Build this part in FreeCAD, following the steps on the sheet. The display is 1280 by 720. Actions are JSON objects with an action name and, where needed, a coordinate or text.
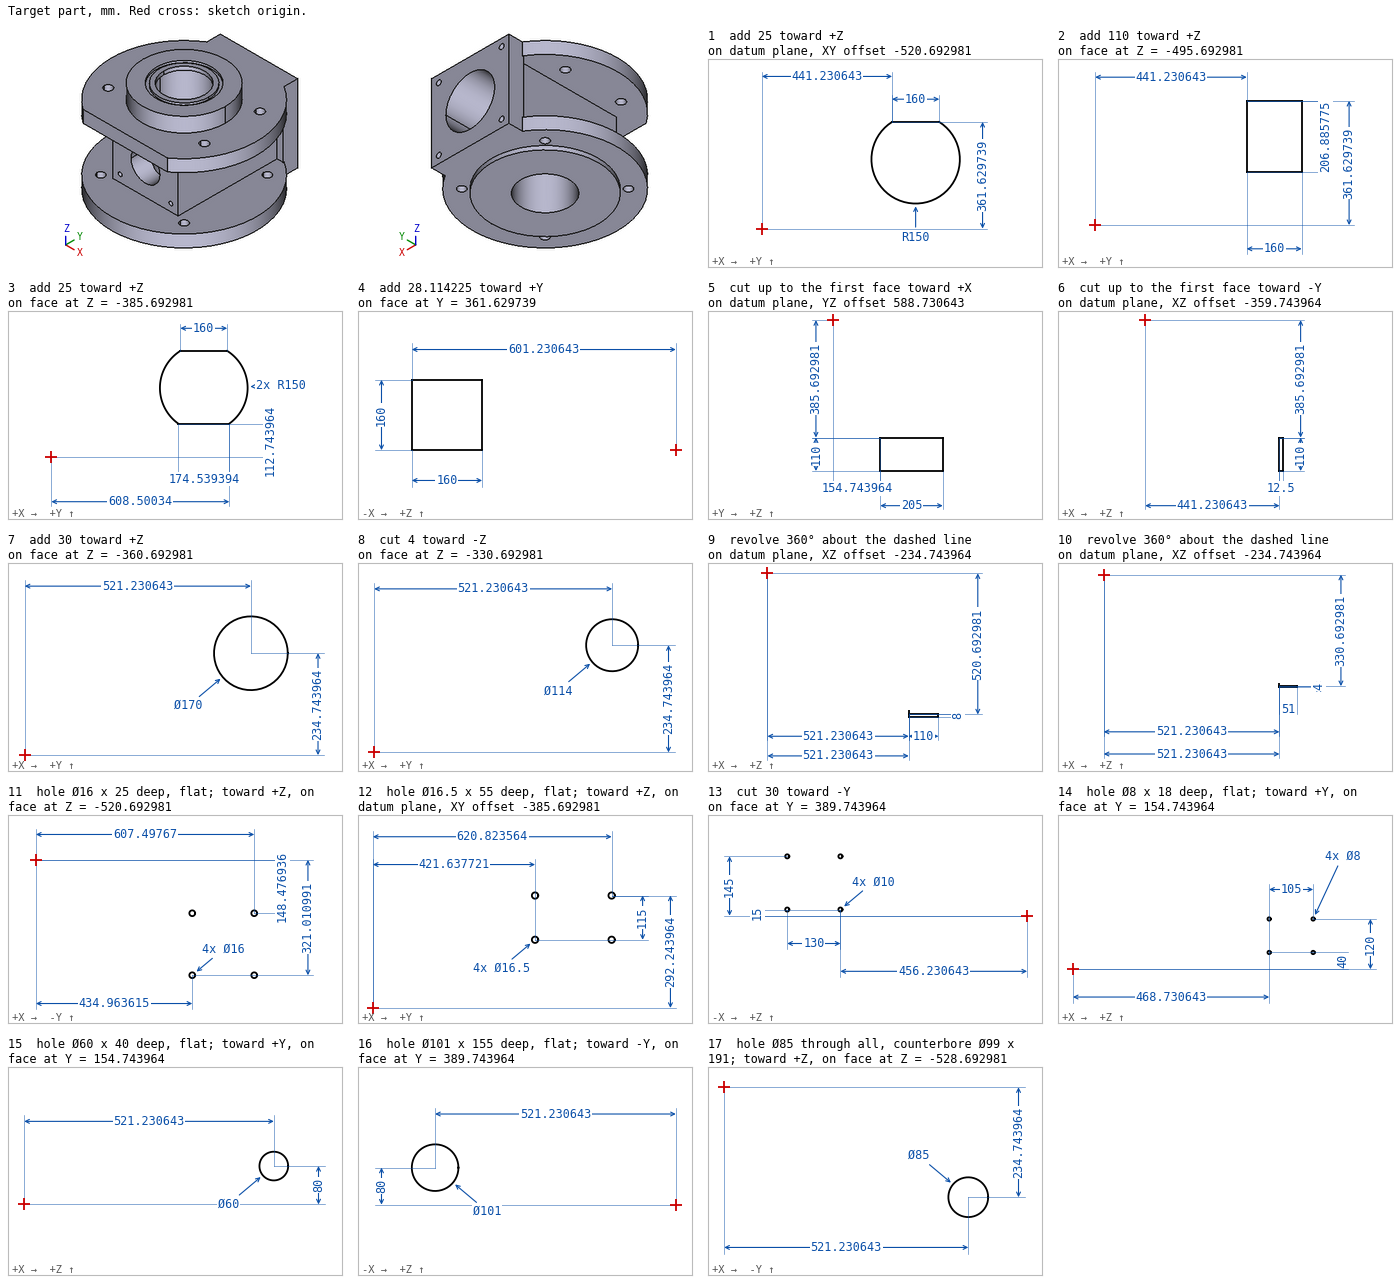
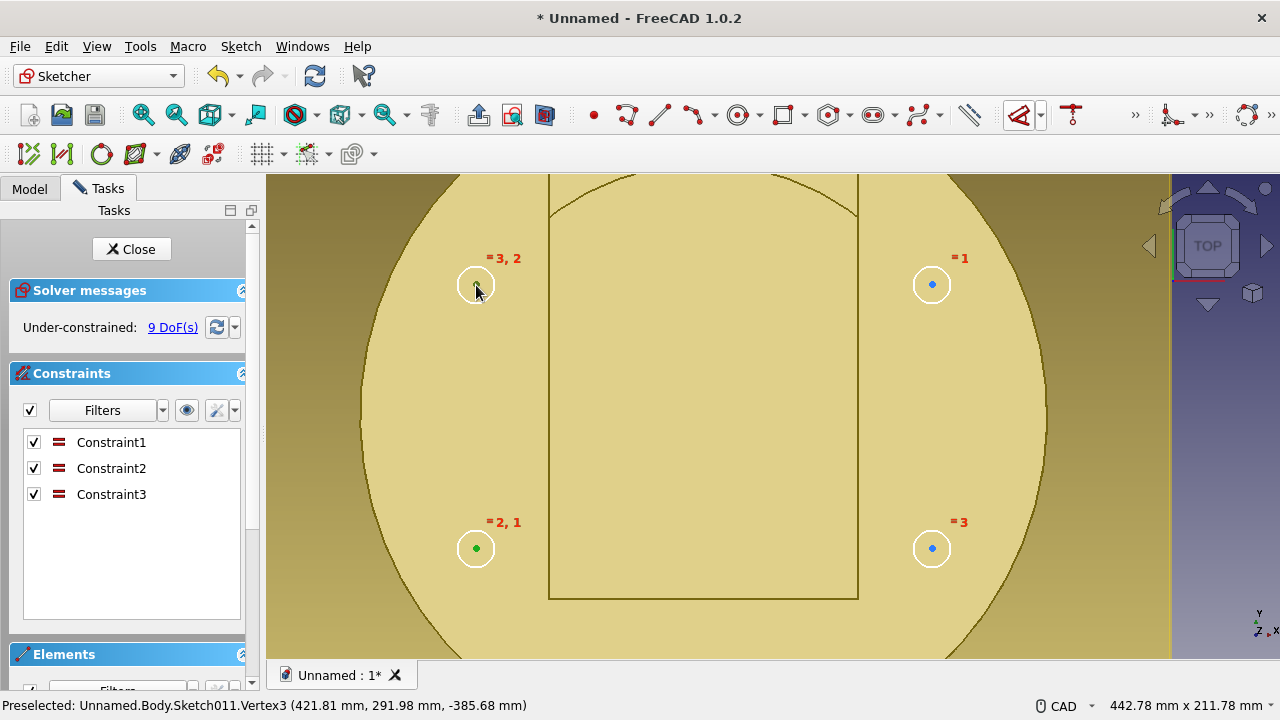
{"action": "key", "text": "v"}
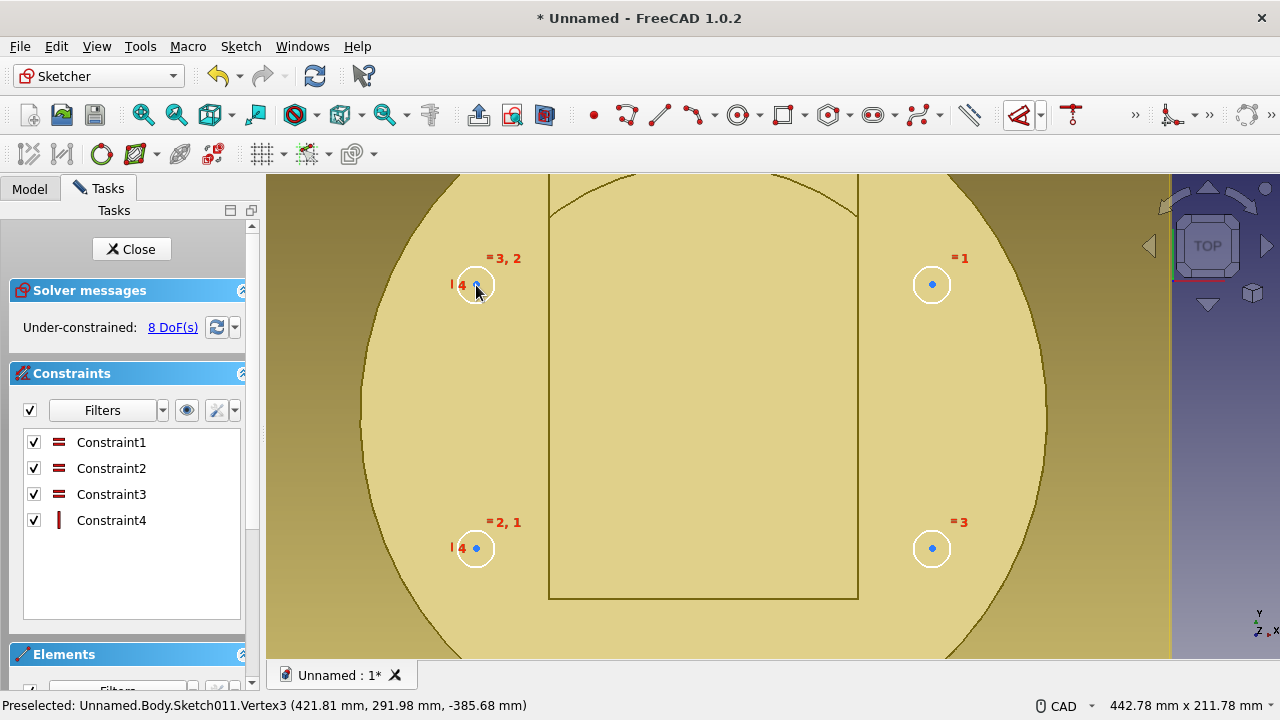
{"action": "left_click", "coordinate": [932, 285]}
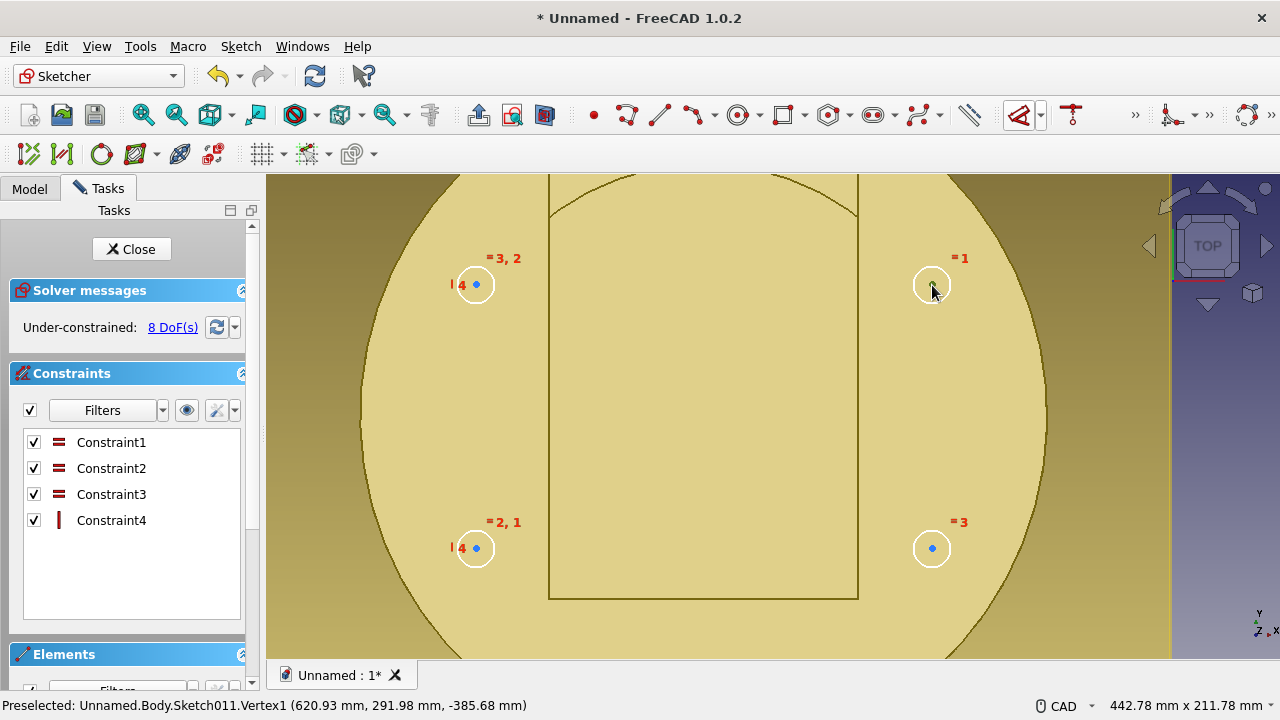
{"action": "left_click", "coordinate": [476, 285]}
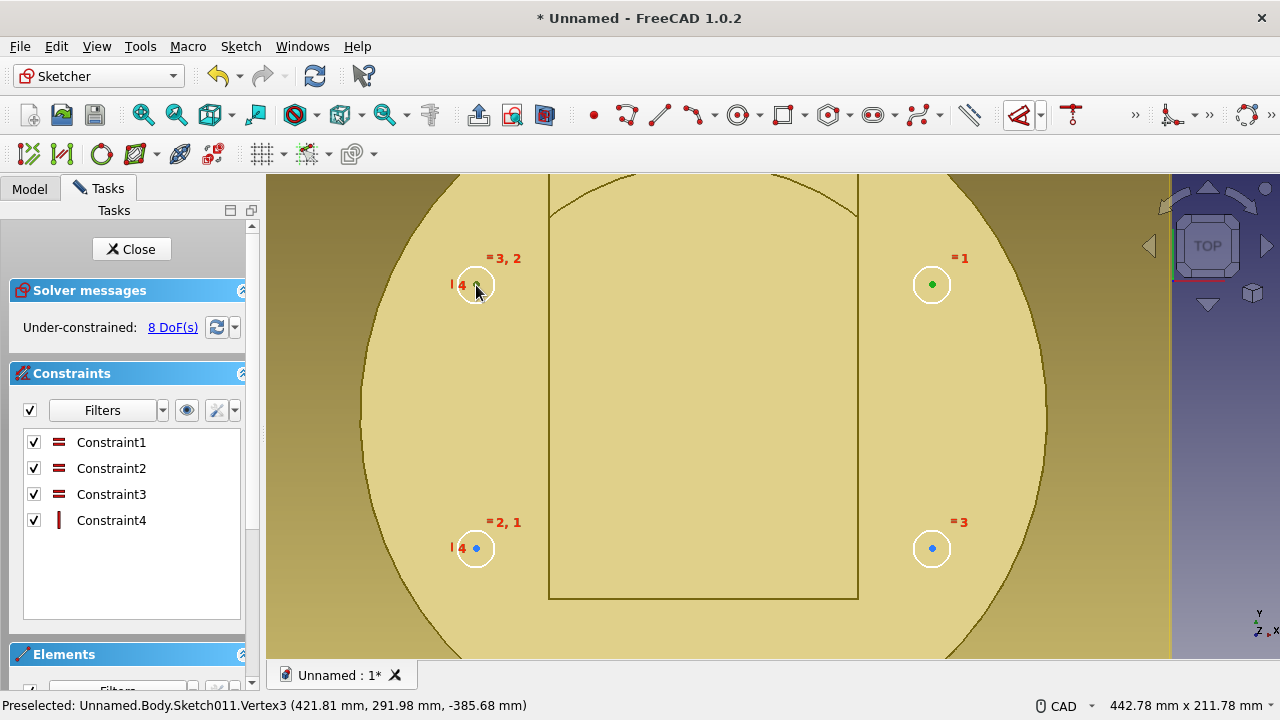
{"action": "key", "text": "h"}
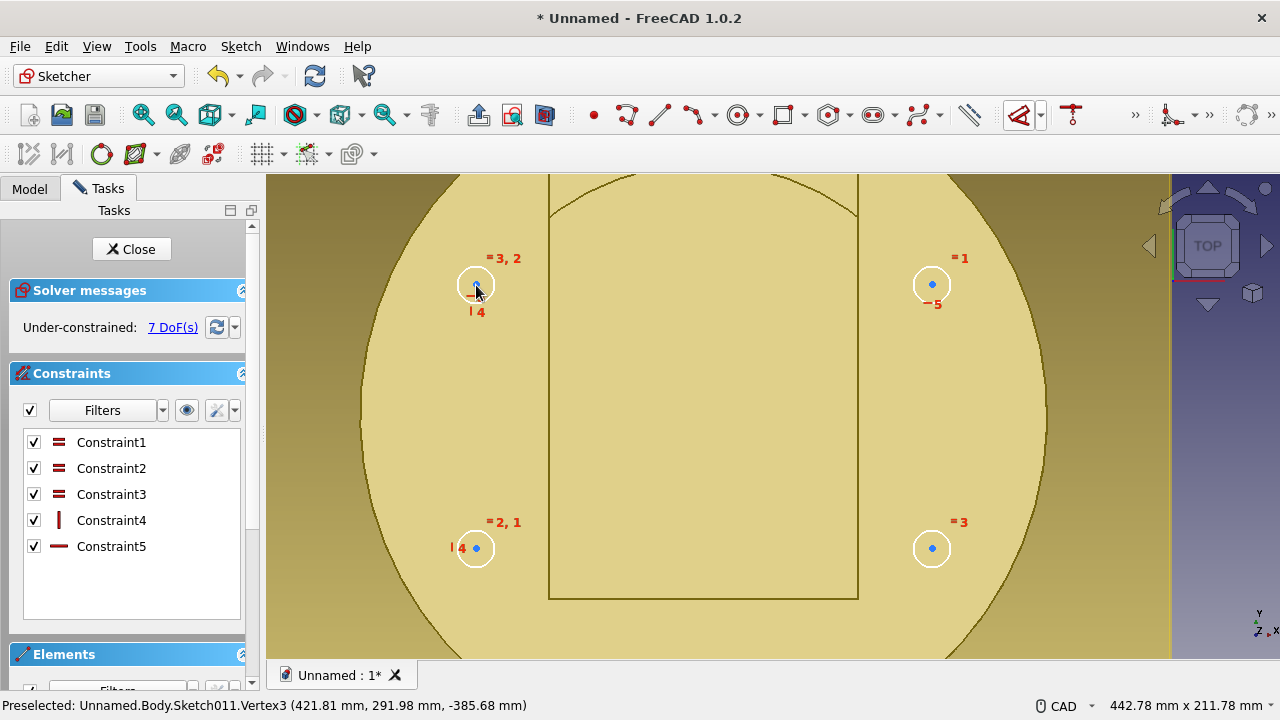
{"action": "left_click", "coordinate": [932, 285]}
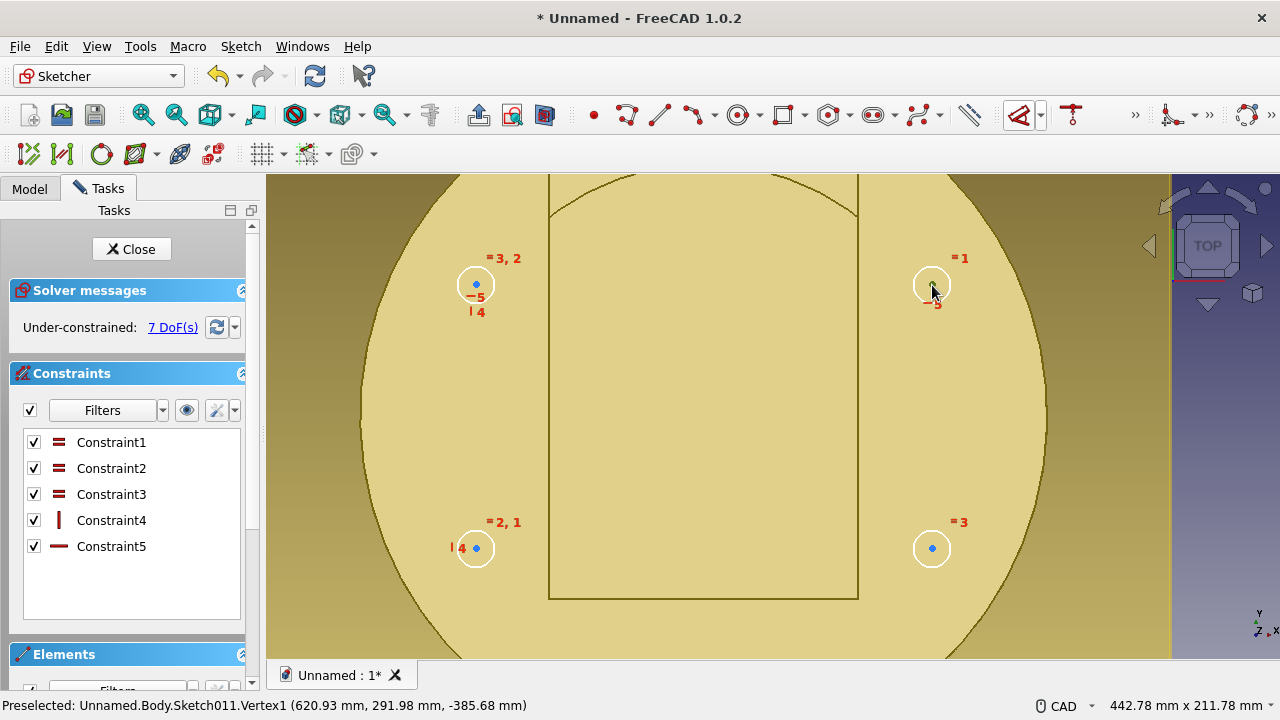
{"action": "left_click", "coordinate": [932, 549]}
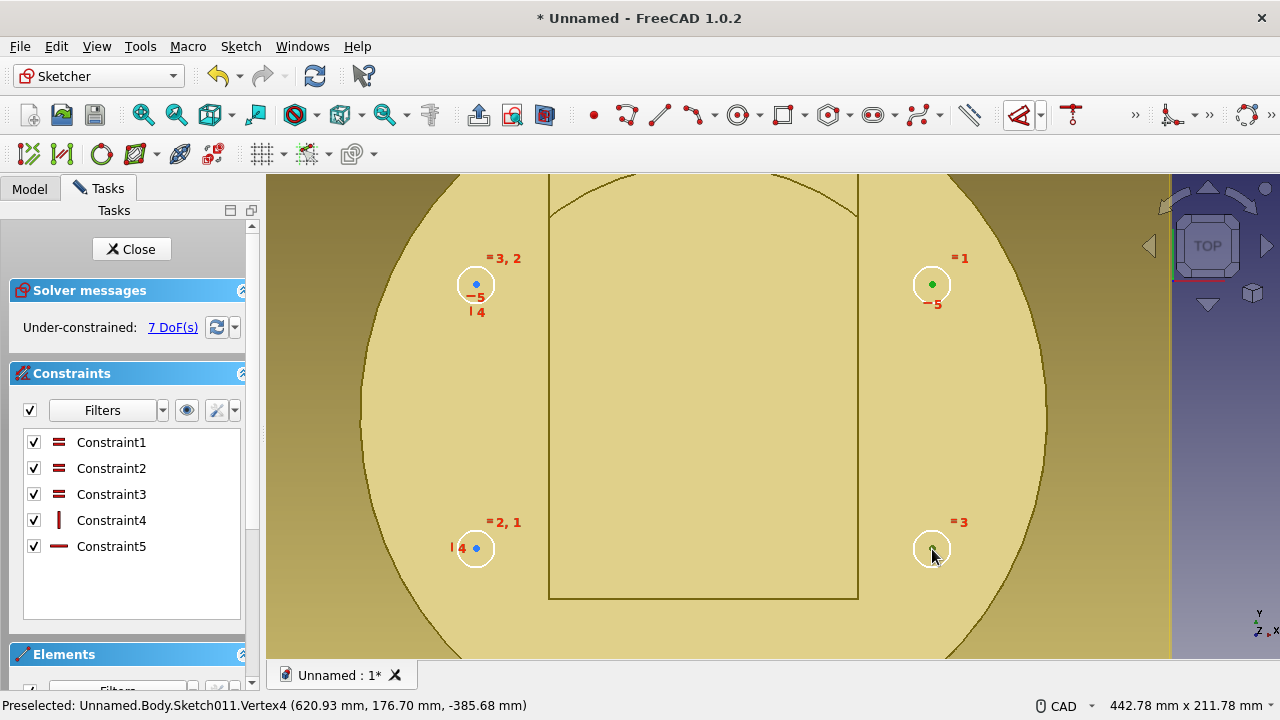
{"action": "key", "text": "v"}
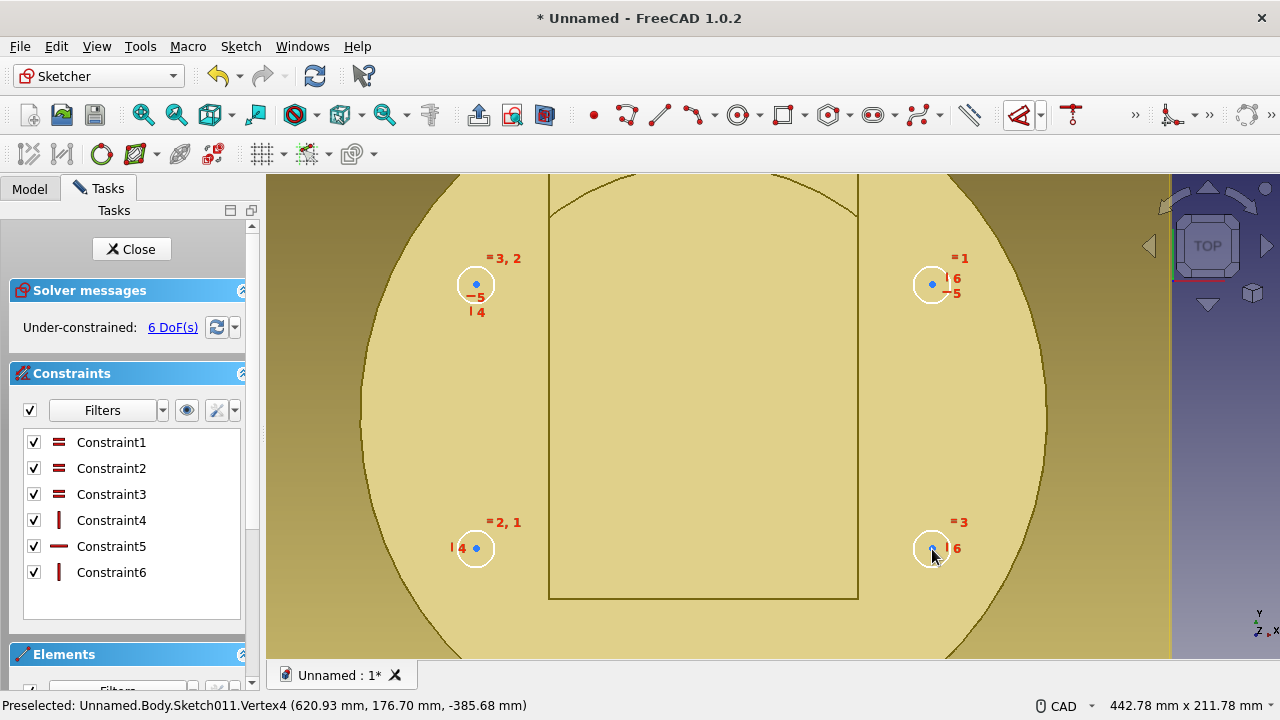
{"action": "left_click", "coordinate": [476, 549]}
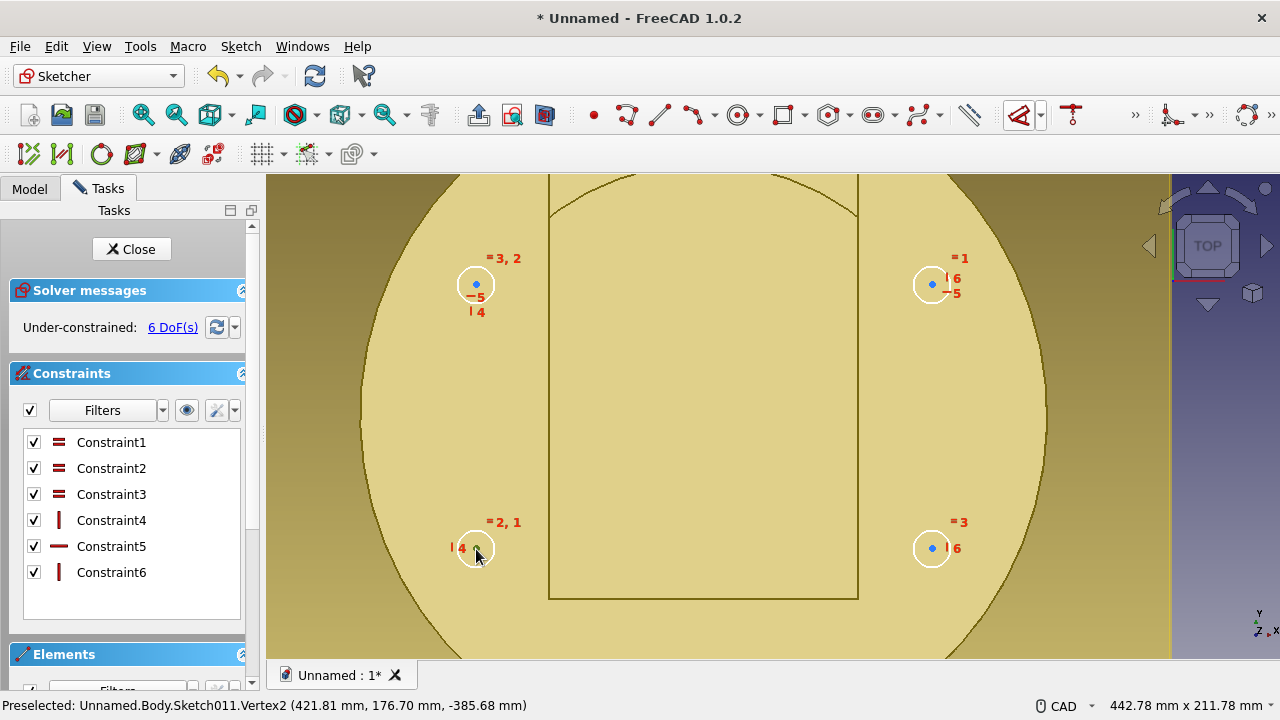
{"action": "left_click", "coordinate": [932, 549]}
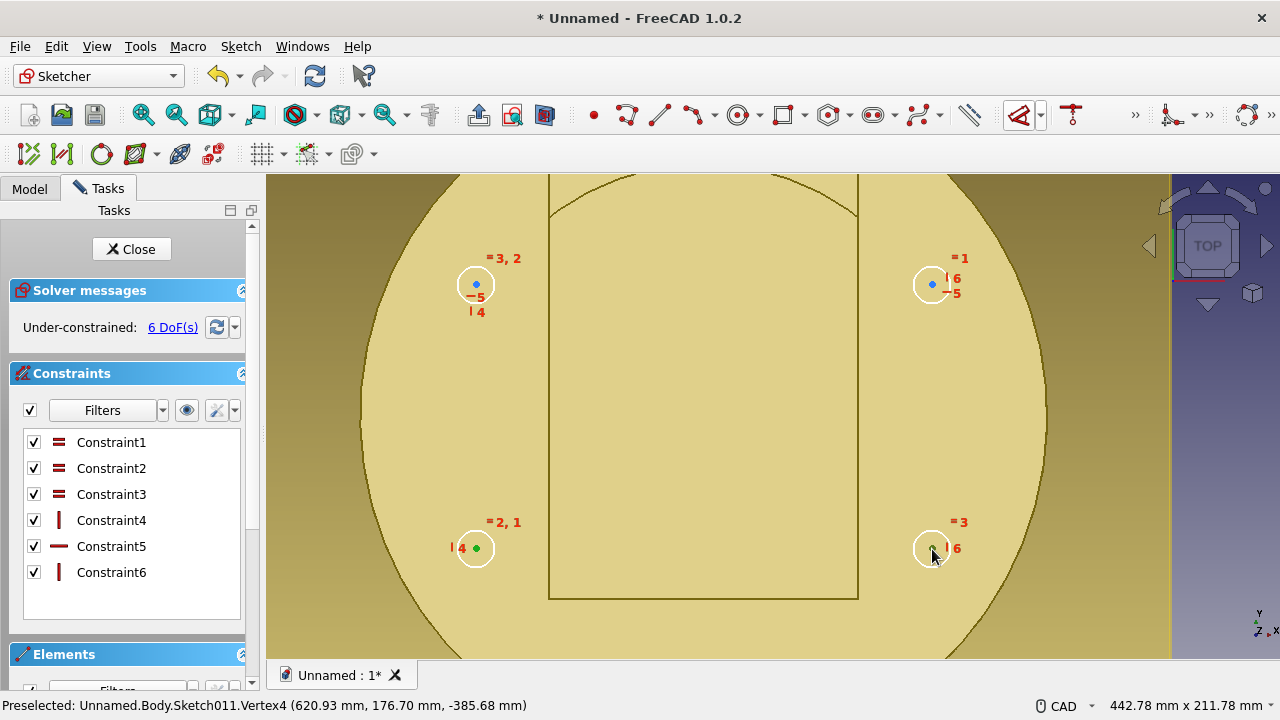
{"action": "key", "text": "h"}